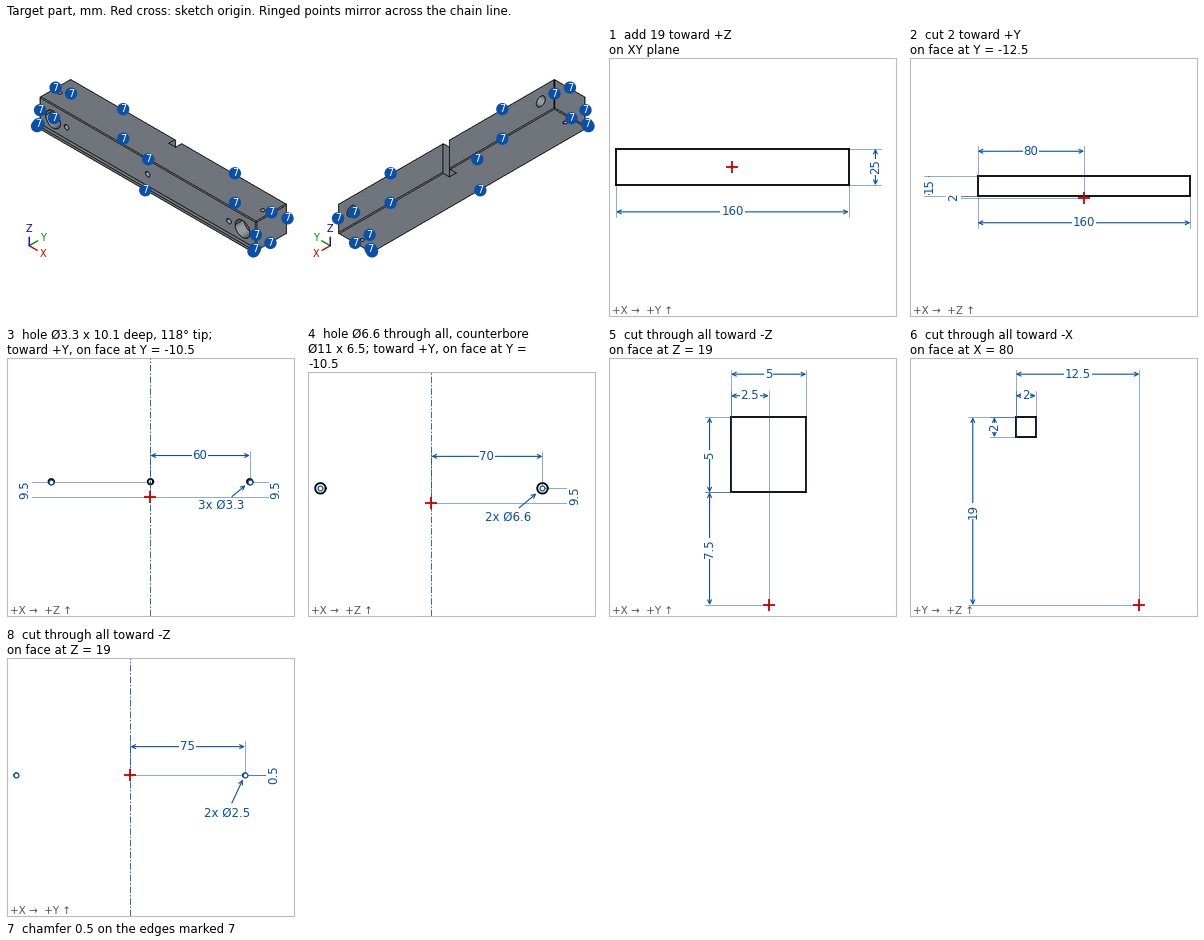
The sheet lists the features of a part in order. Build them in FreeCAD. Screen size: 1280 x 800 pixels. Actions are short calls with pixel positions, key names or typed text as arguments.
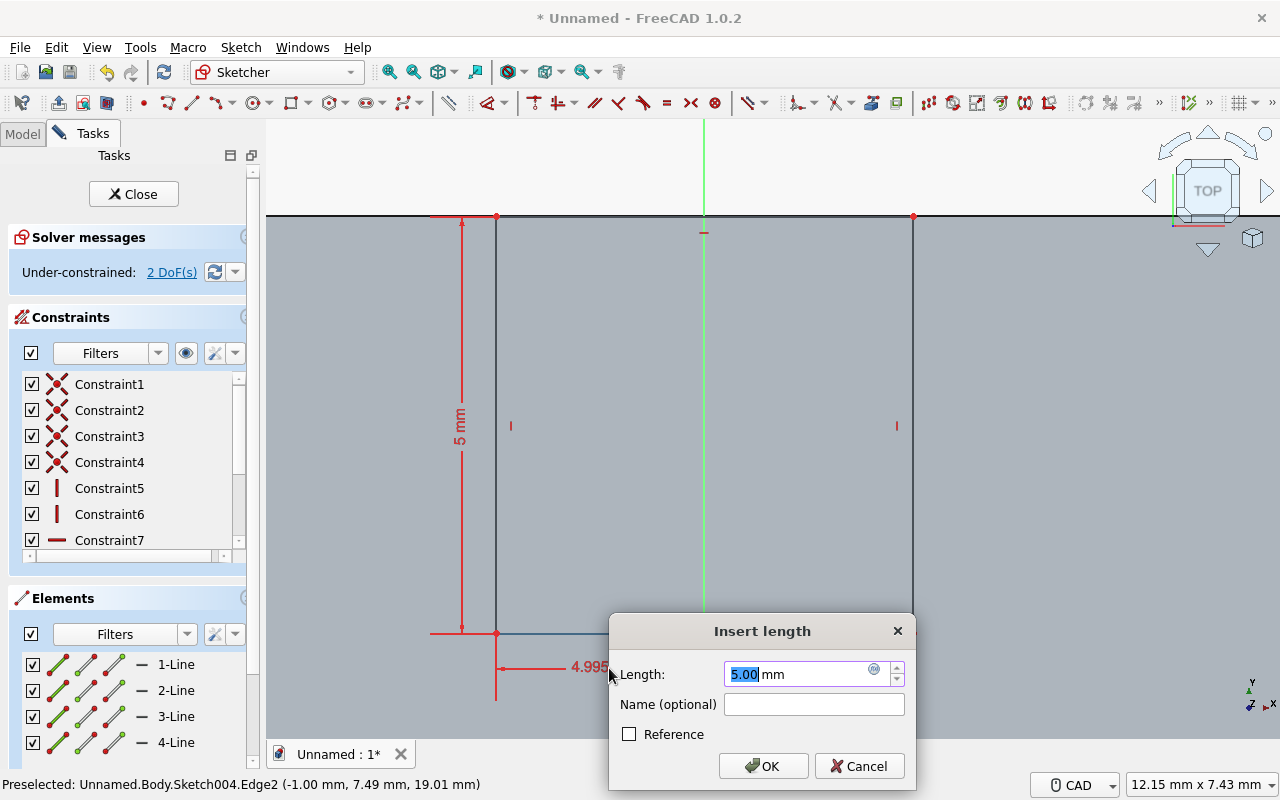
text(5)
key(Return)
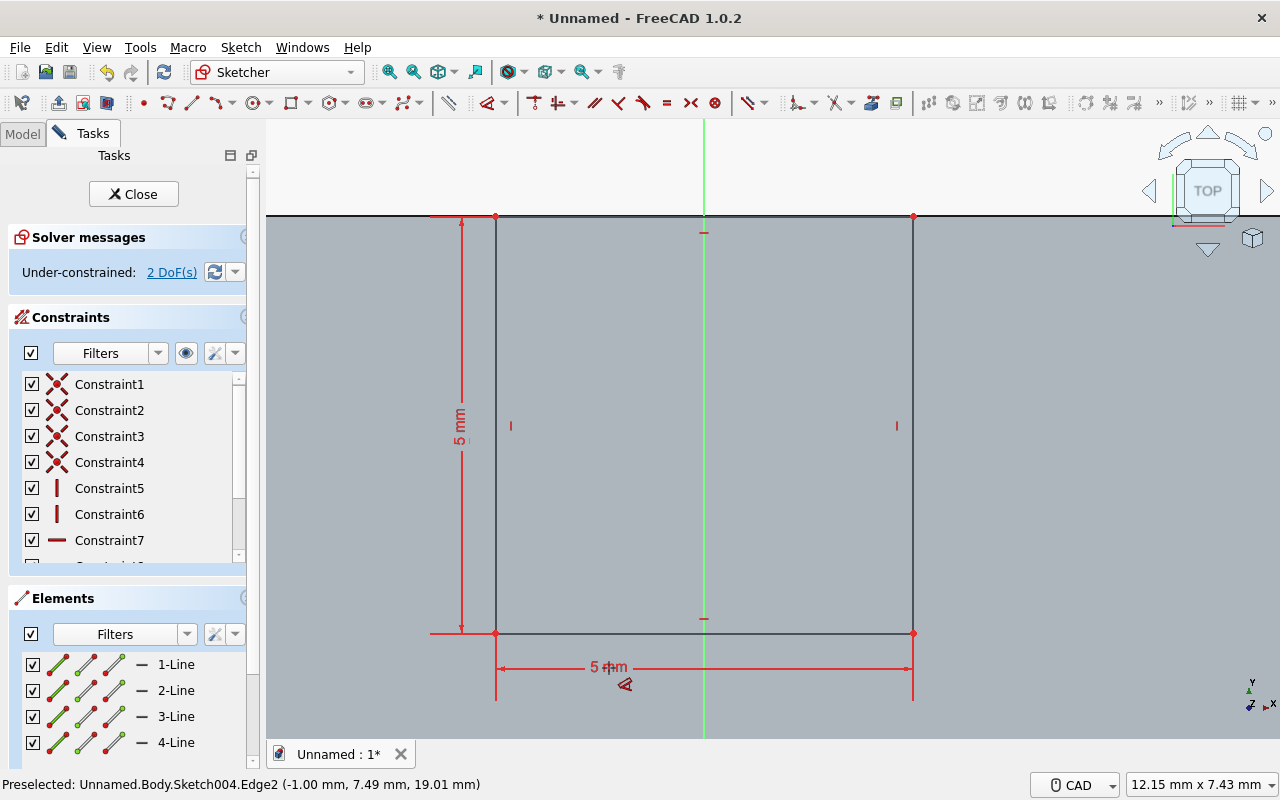
click(496, 217)
click(600, 183)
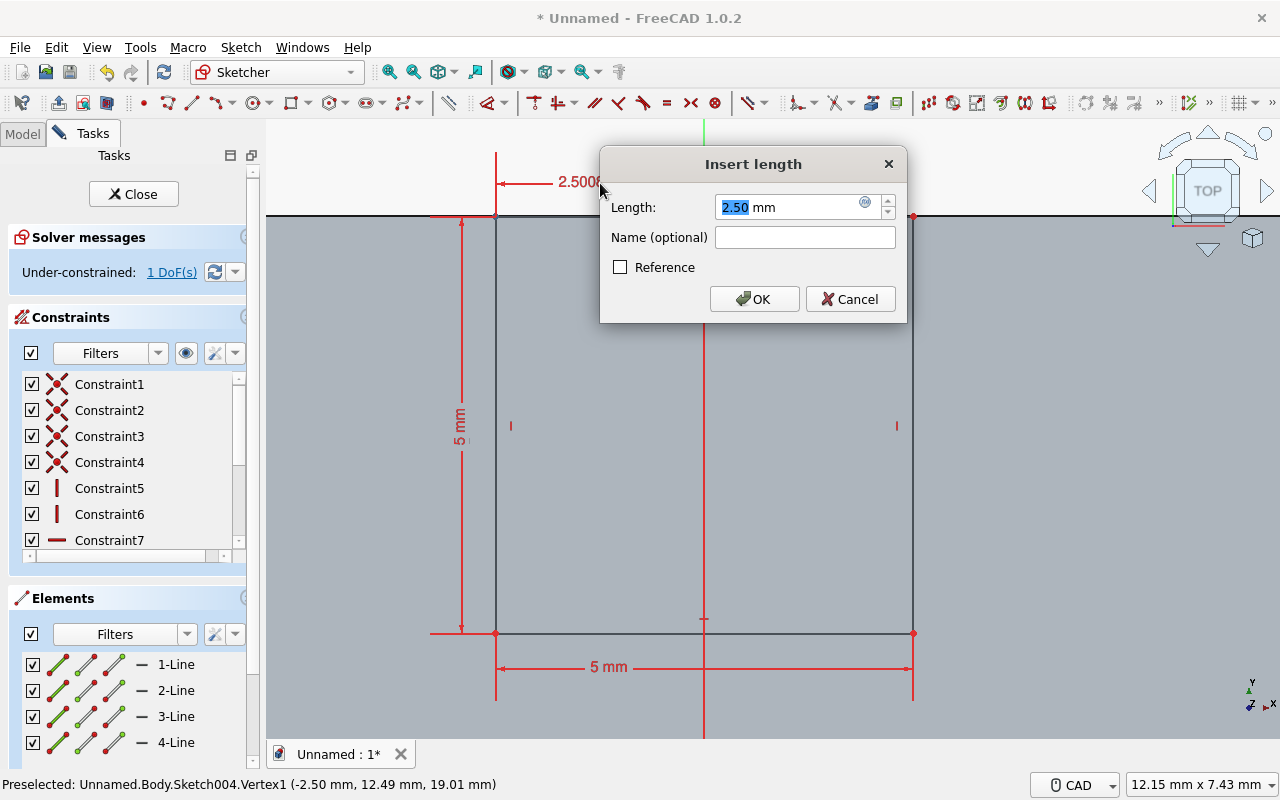
text(2.5)
key(Return)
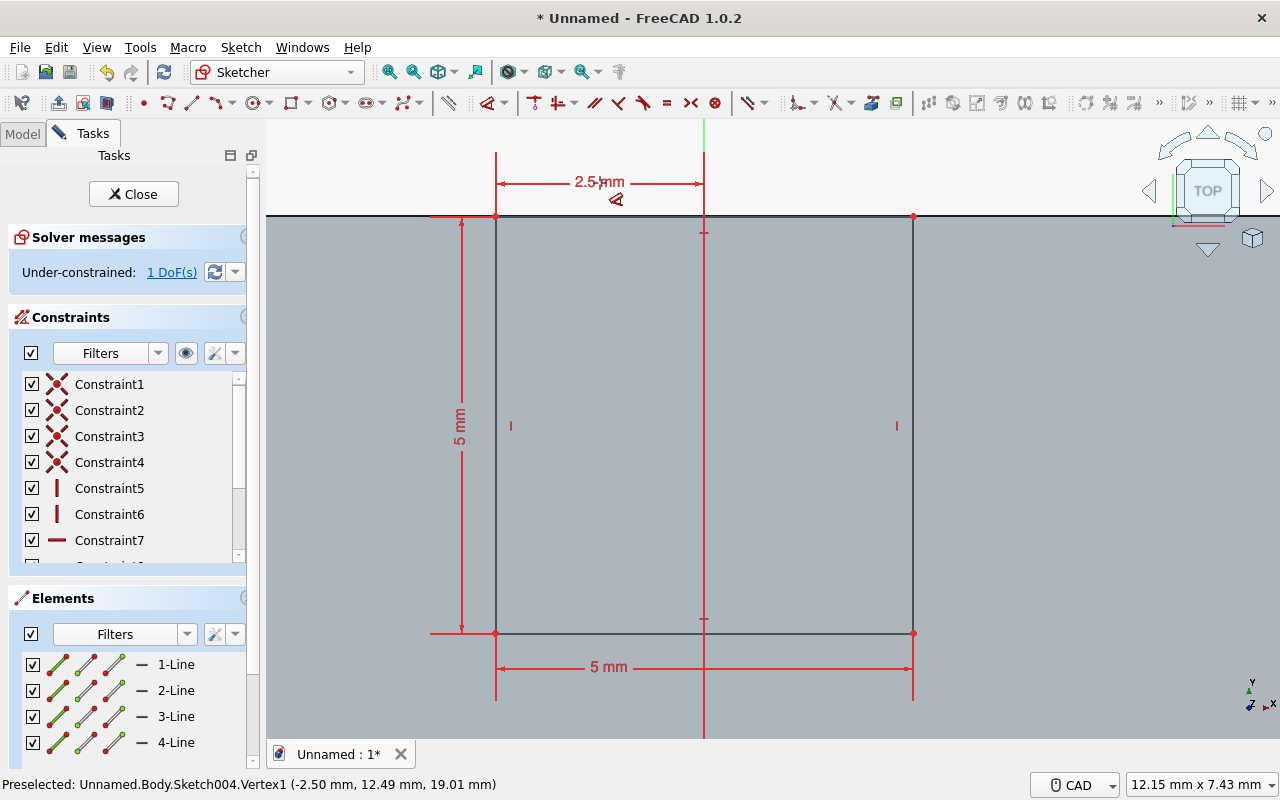
click(496, 634)
click(462, 673)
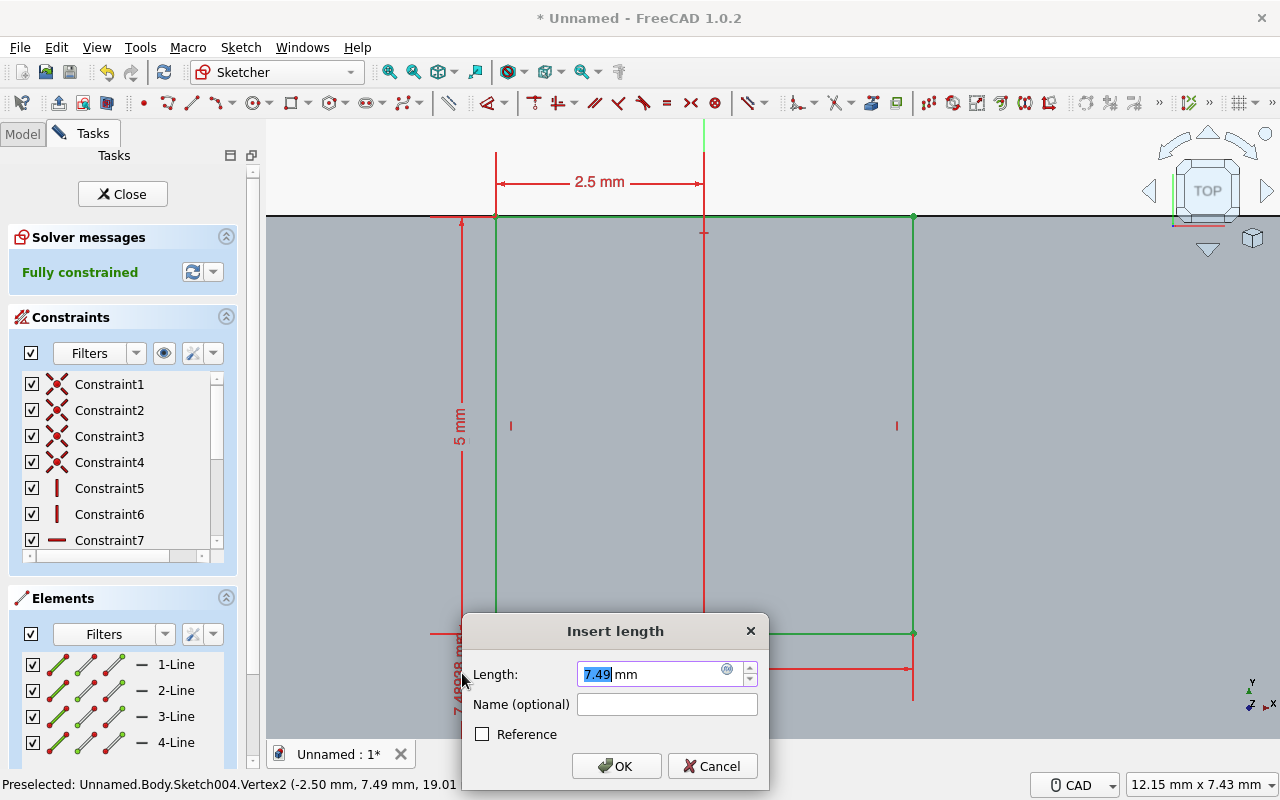
text(7.5)
key(Return)
key(Escape)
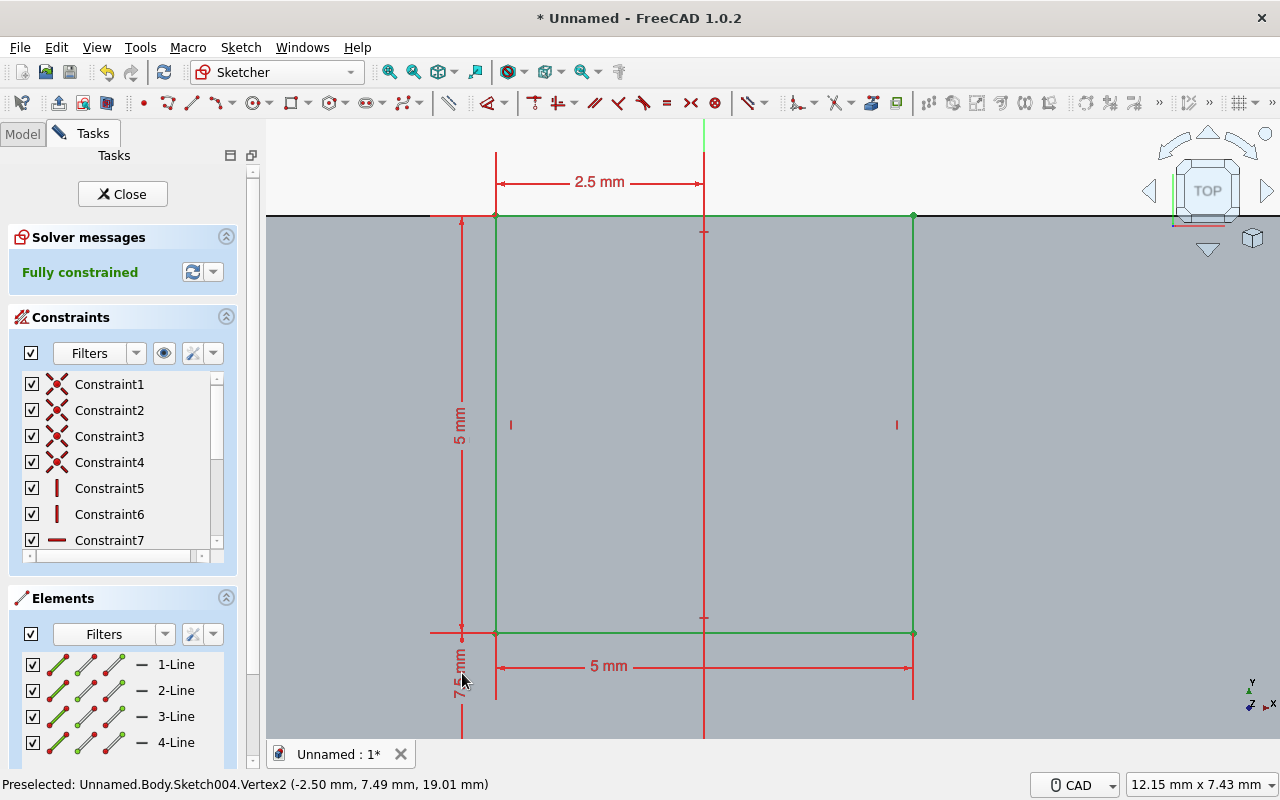
click(123, 194)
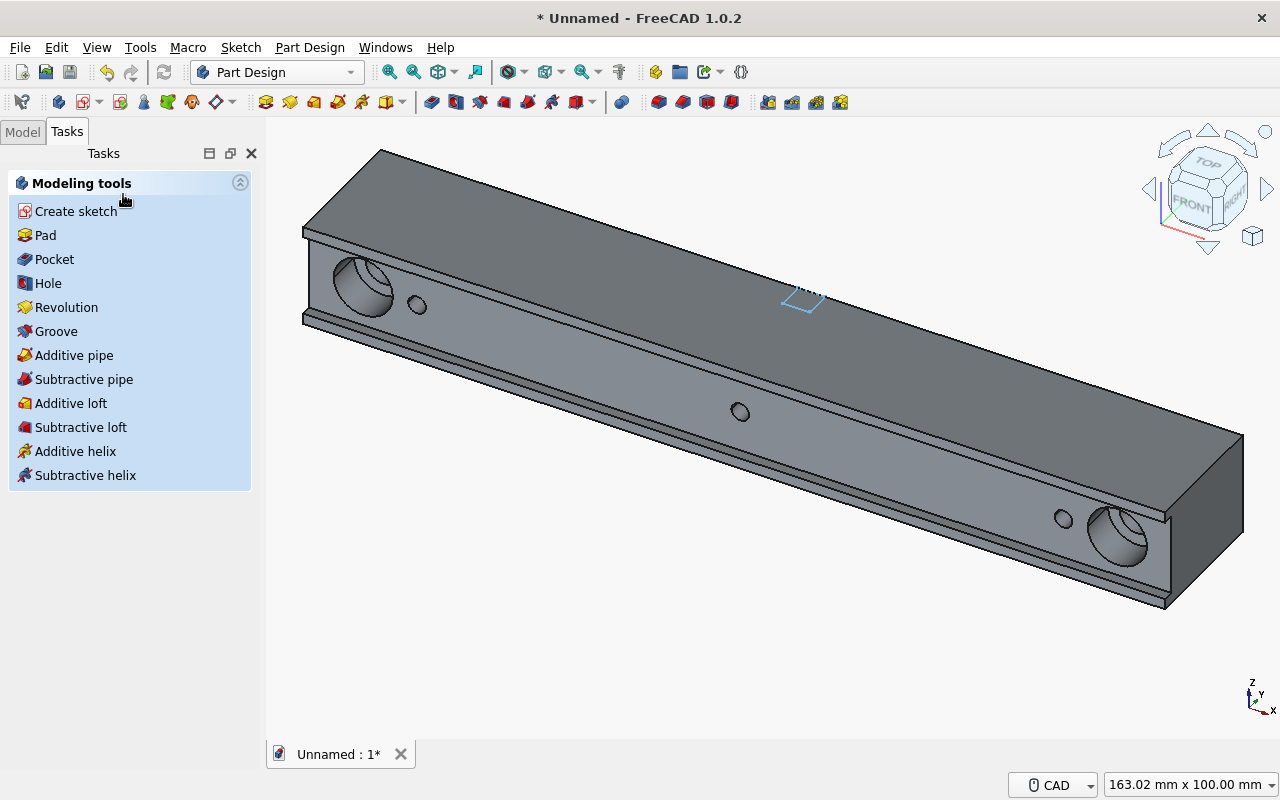
click(432, 102)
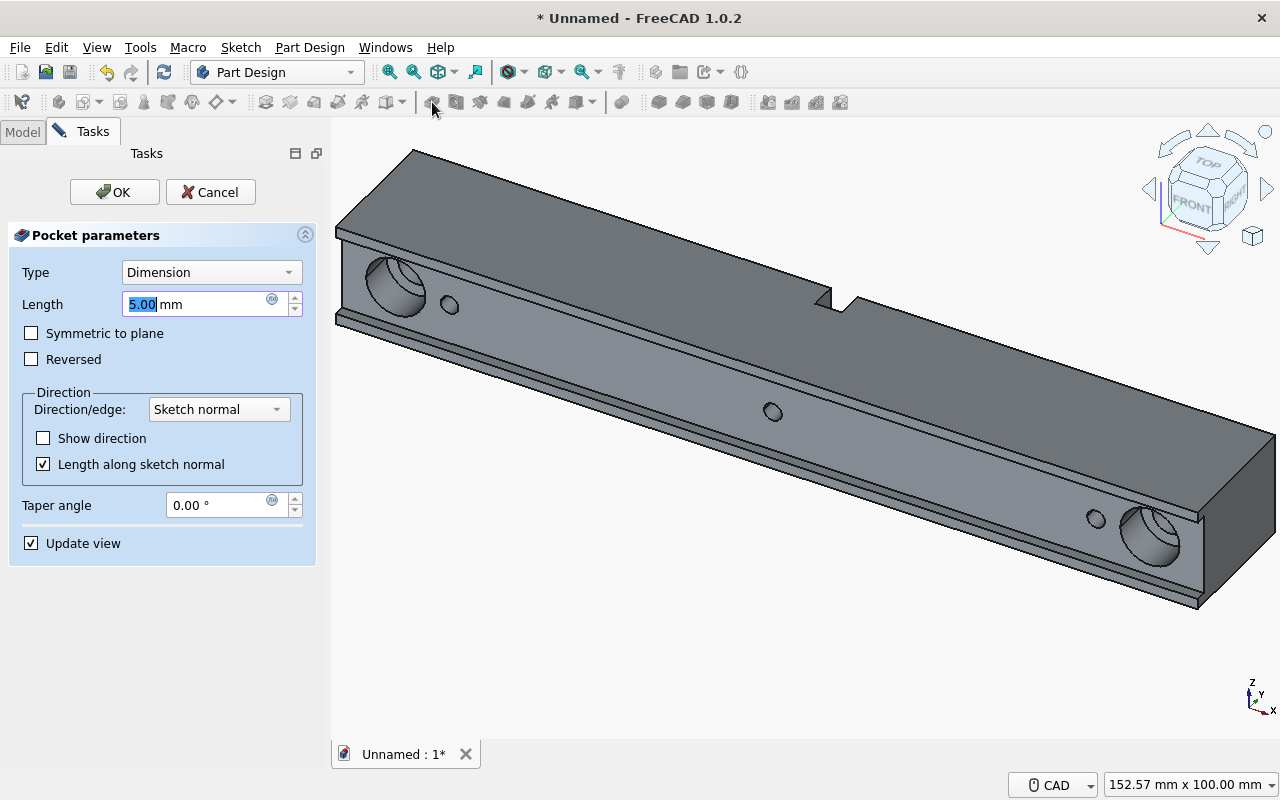
click(212, 272)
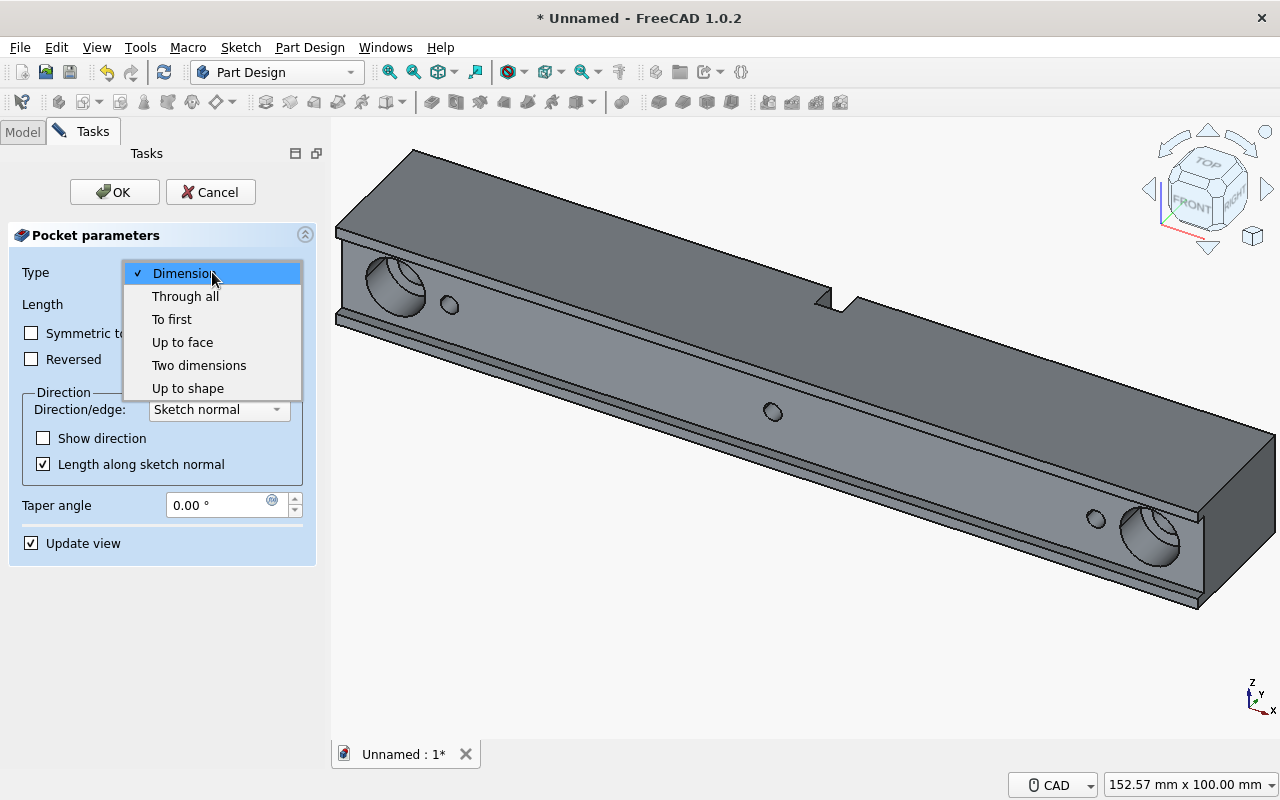
click(212, 296)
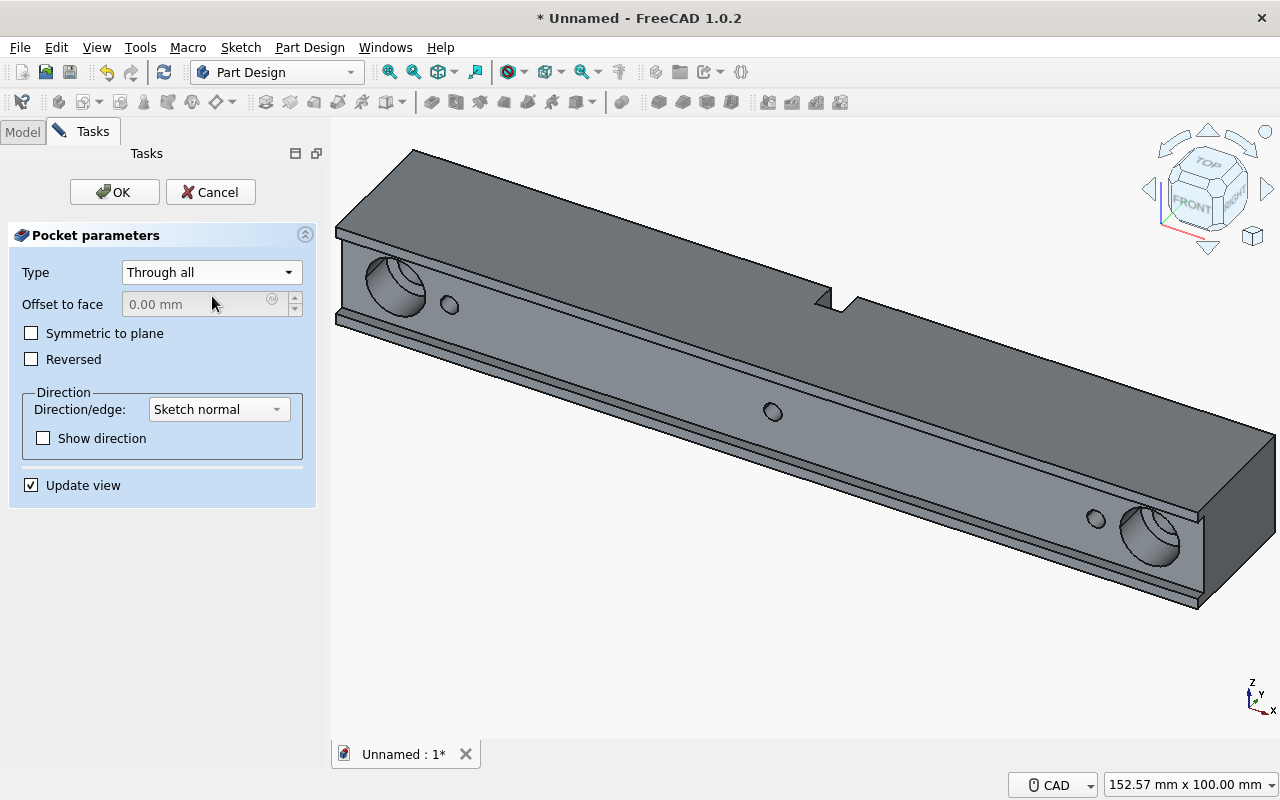
click(115, 192)